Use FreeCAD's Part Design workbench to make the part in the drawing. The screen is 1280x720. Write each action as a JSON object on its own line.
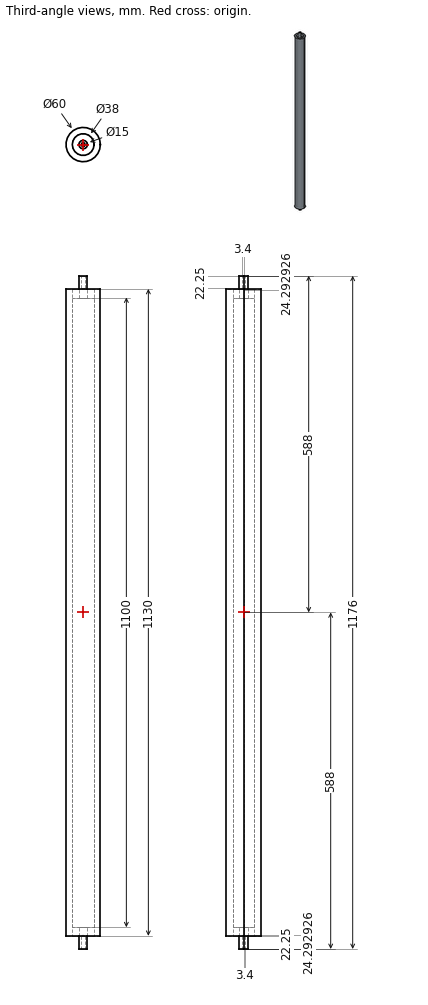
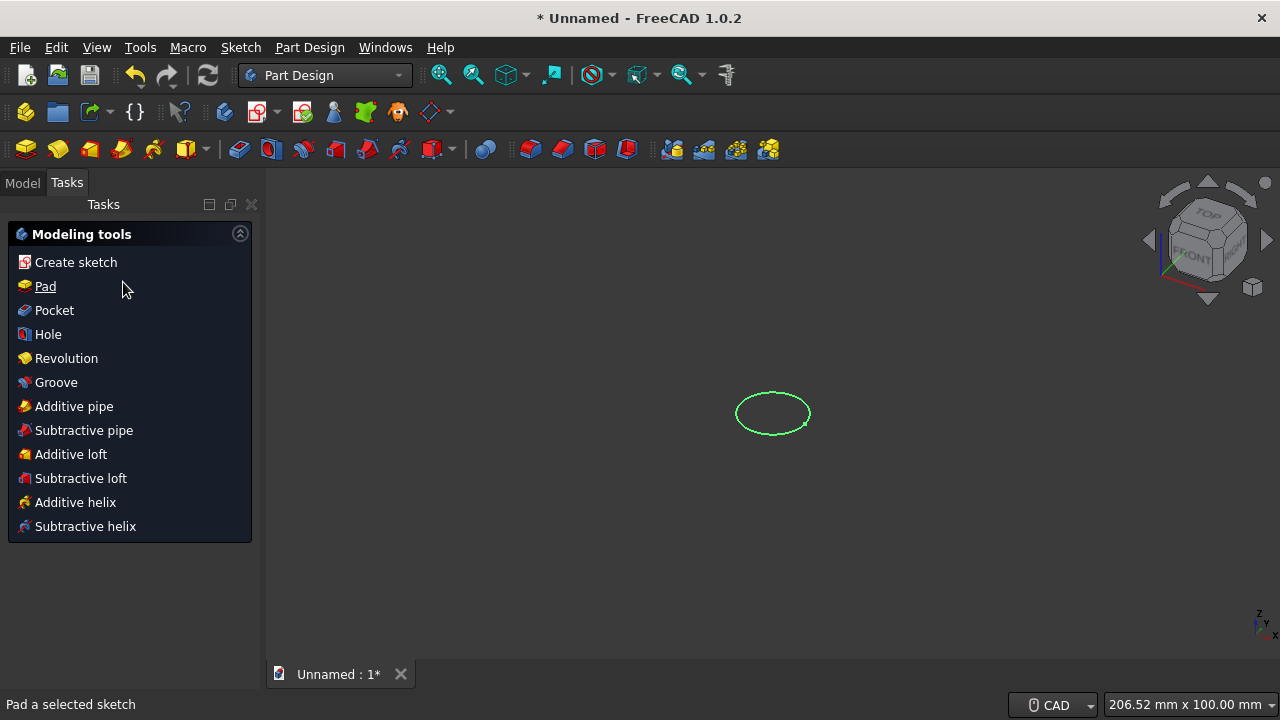
{"action": "left_click", "coordinate": [26, 150]}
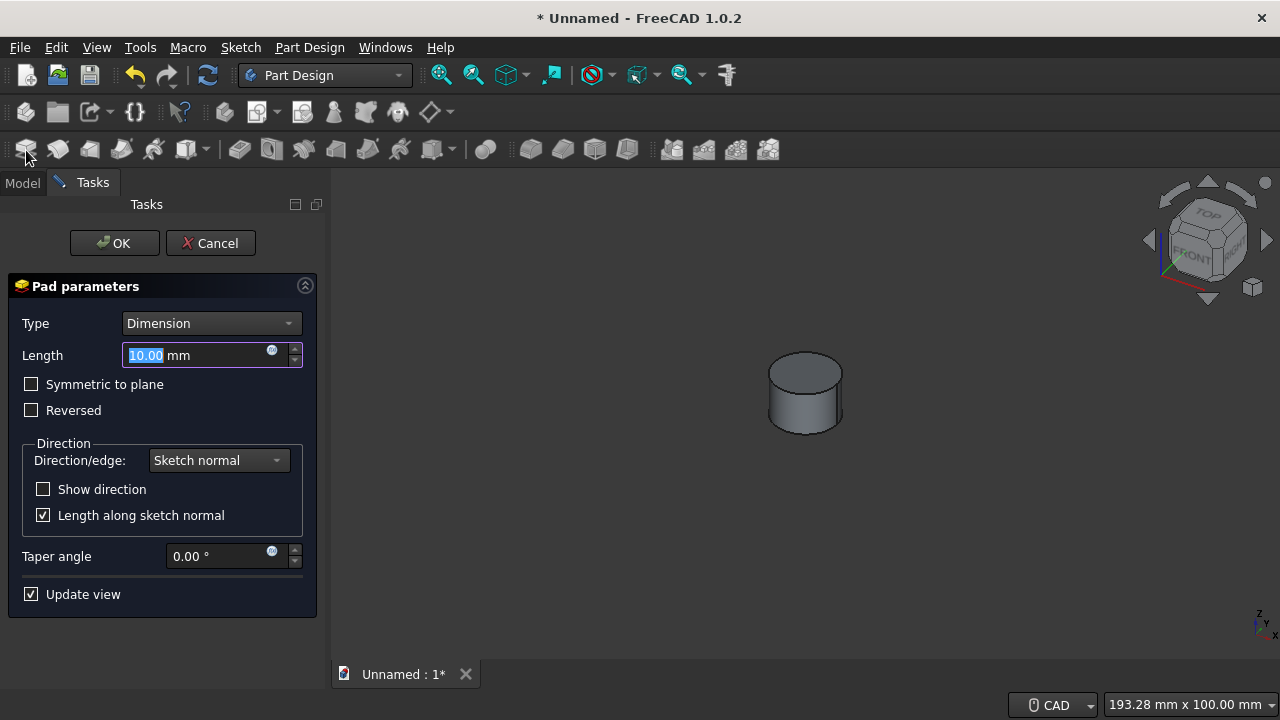
{"action": "type", "text": "1176"}
{"action": "key", "text": "Tab"}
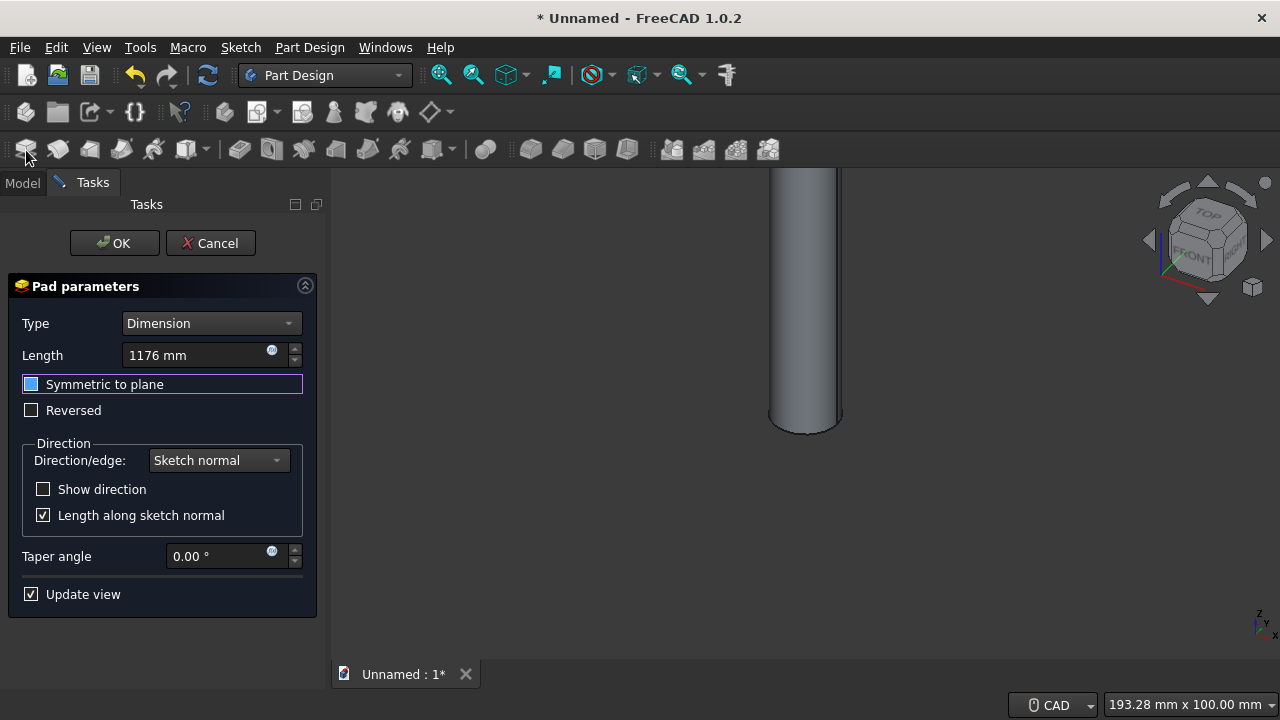
{"action": "left_click", "coordinate": [30, 384]}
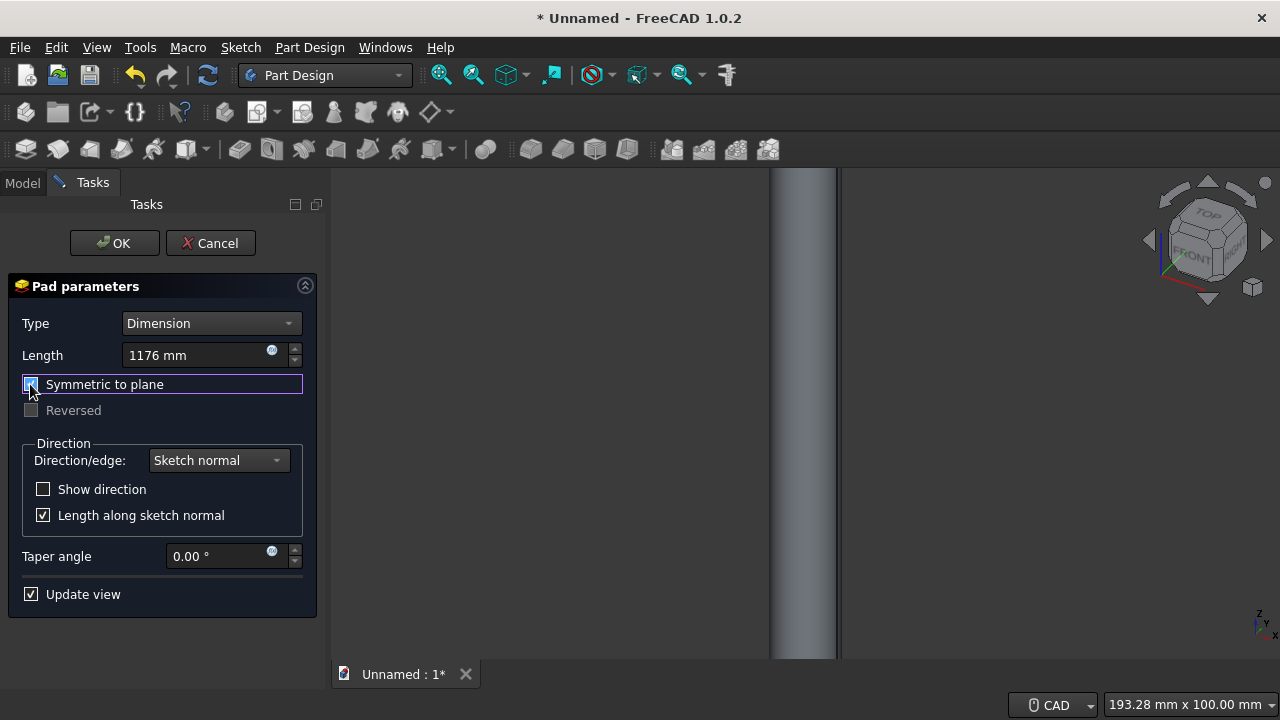
{"action": "left_click", "coordinate": [115, 243]}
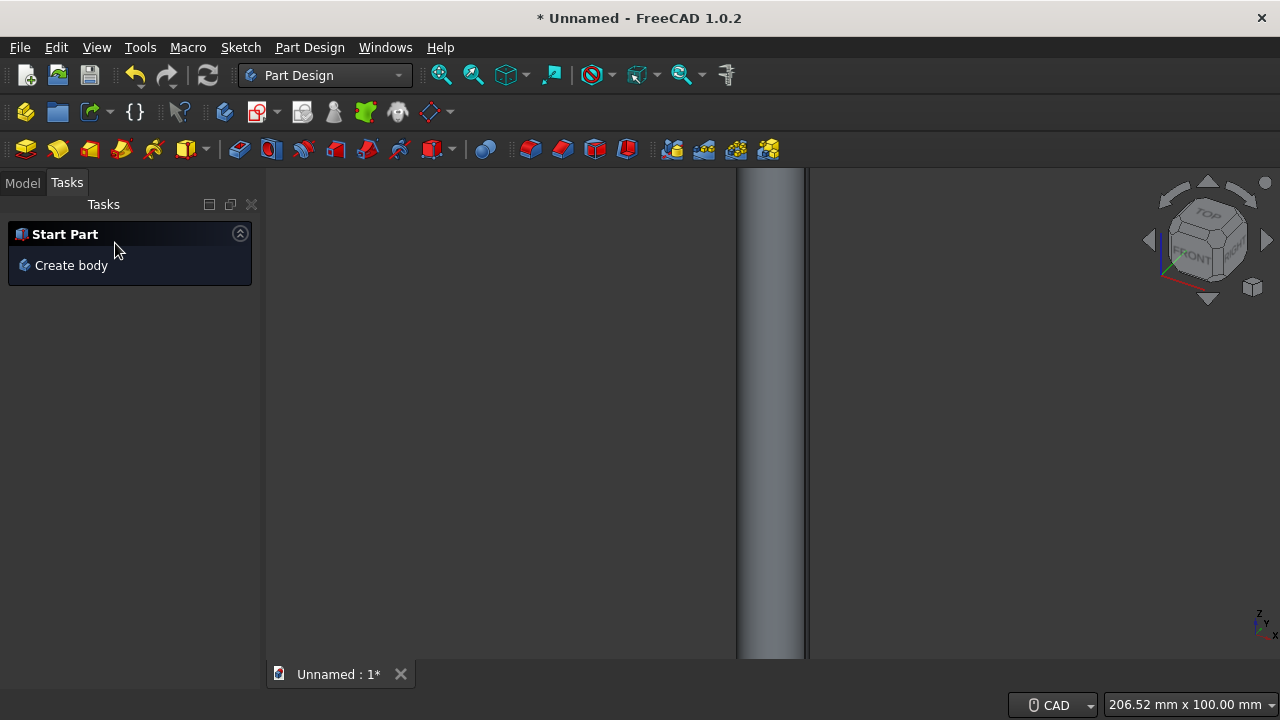
{"action": "left_click", "coordinate": [442, 76]}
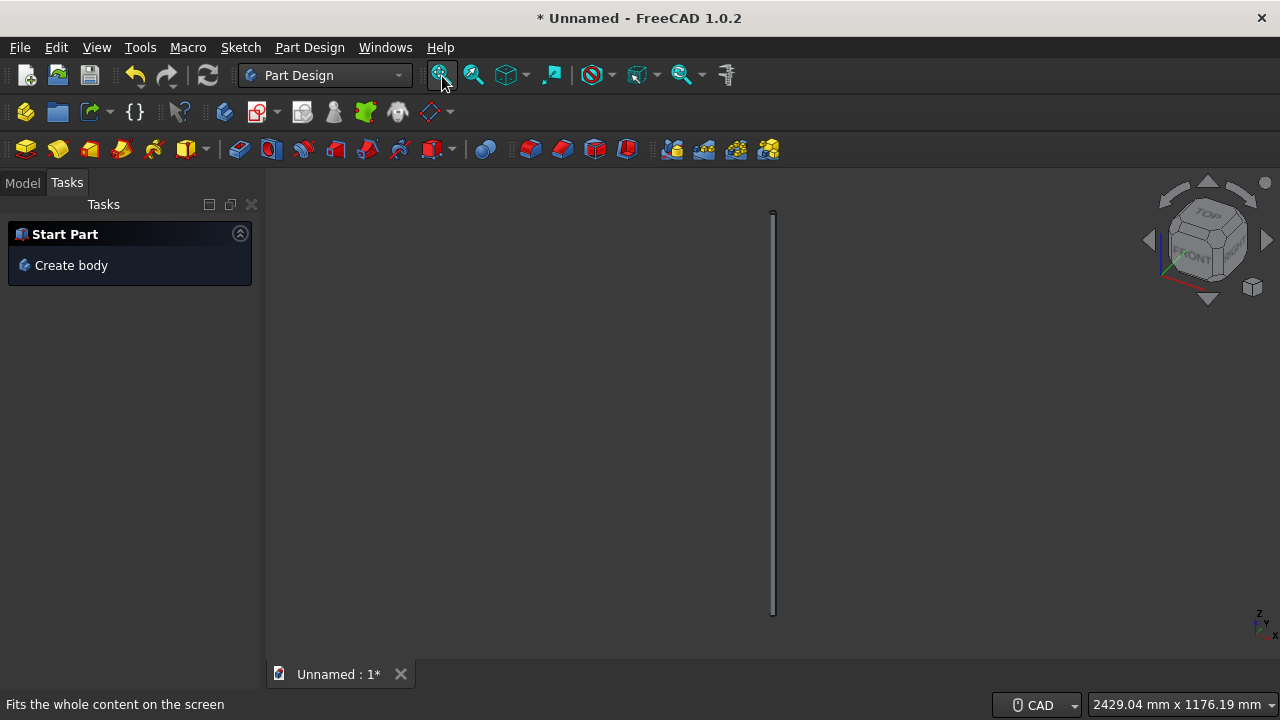
{"action": "left_click", "coordinate": [258, 112]}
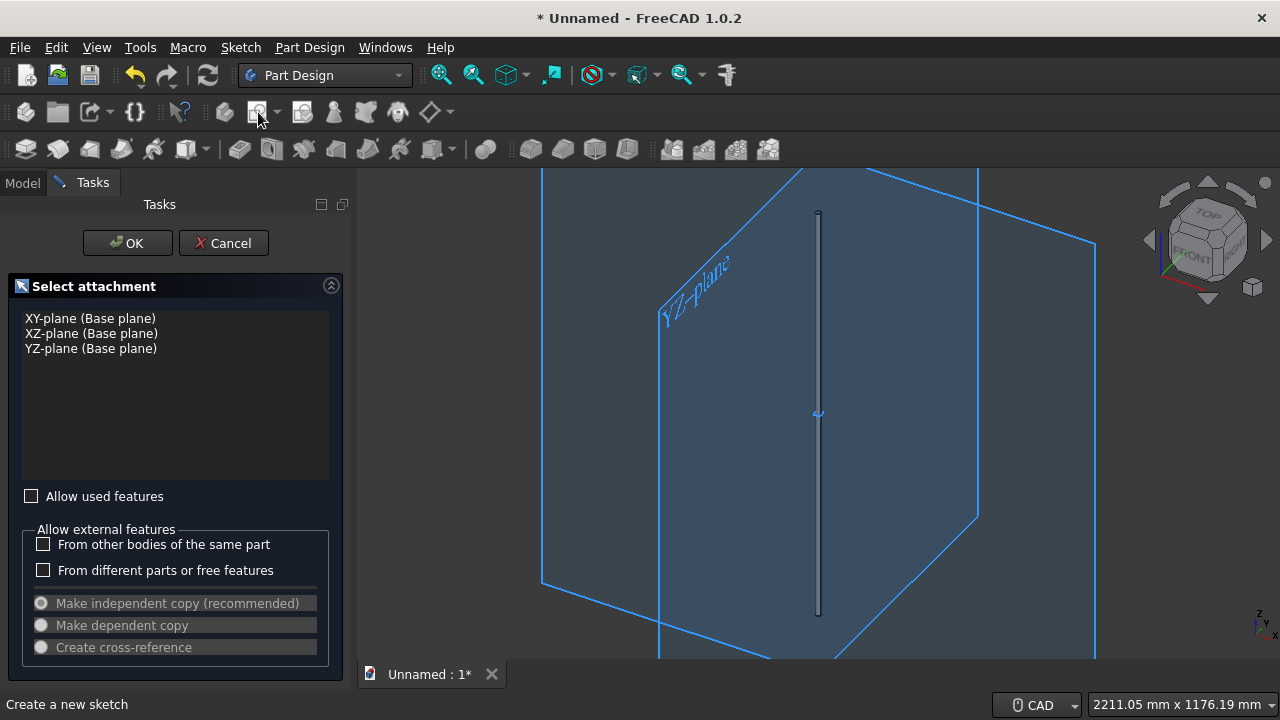
{"action": "left_click", "coordinate": [82, 318]}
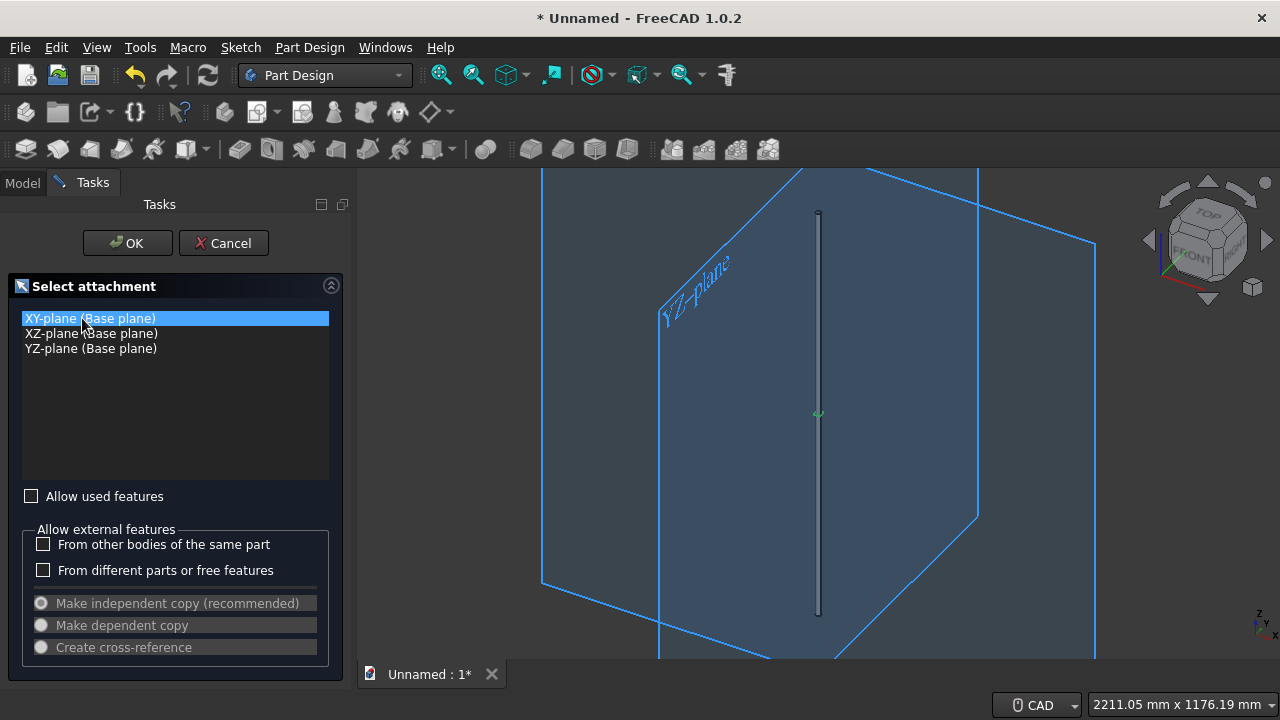
{"action": "left_click", "coordinate": [128, 243]}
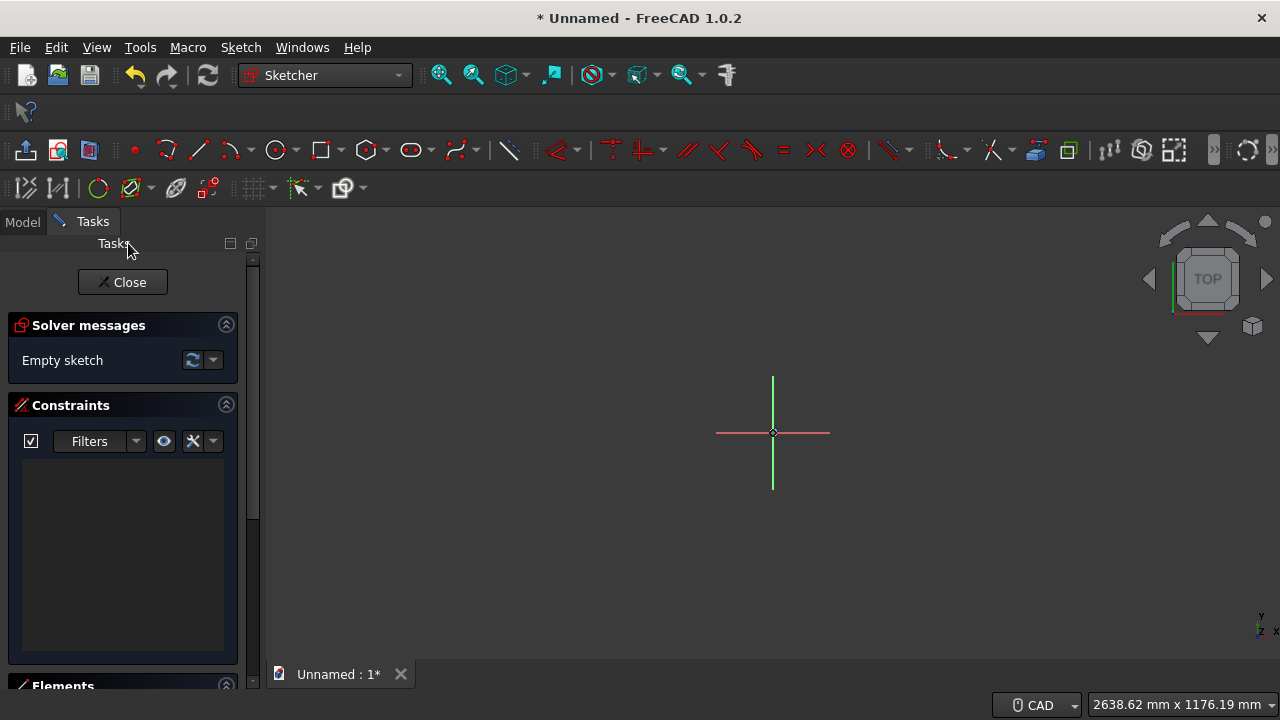
{"action": "left_click", "coordinate": [90, 150]}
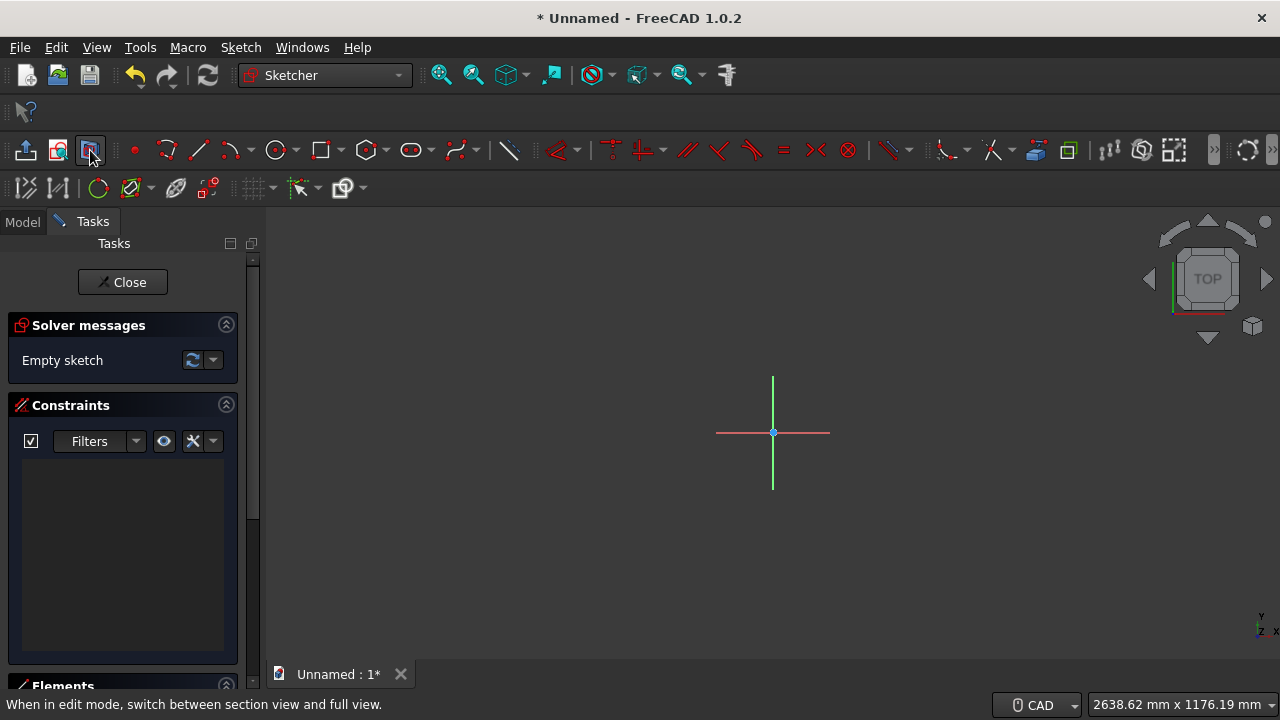
{"action": "scroll", "coordinate": [777, 433], "scroll_direction": "up", "scroll_amount": 15}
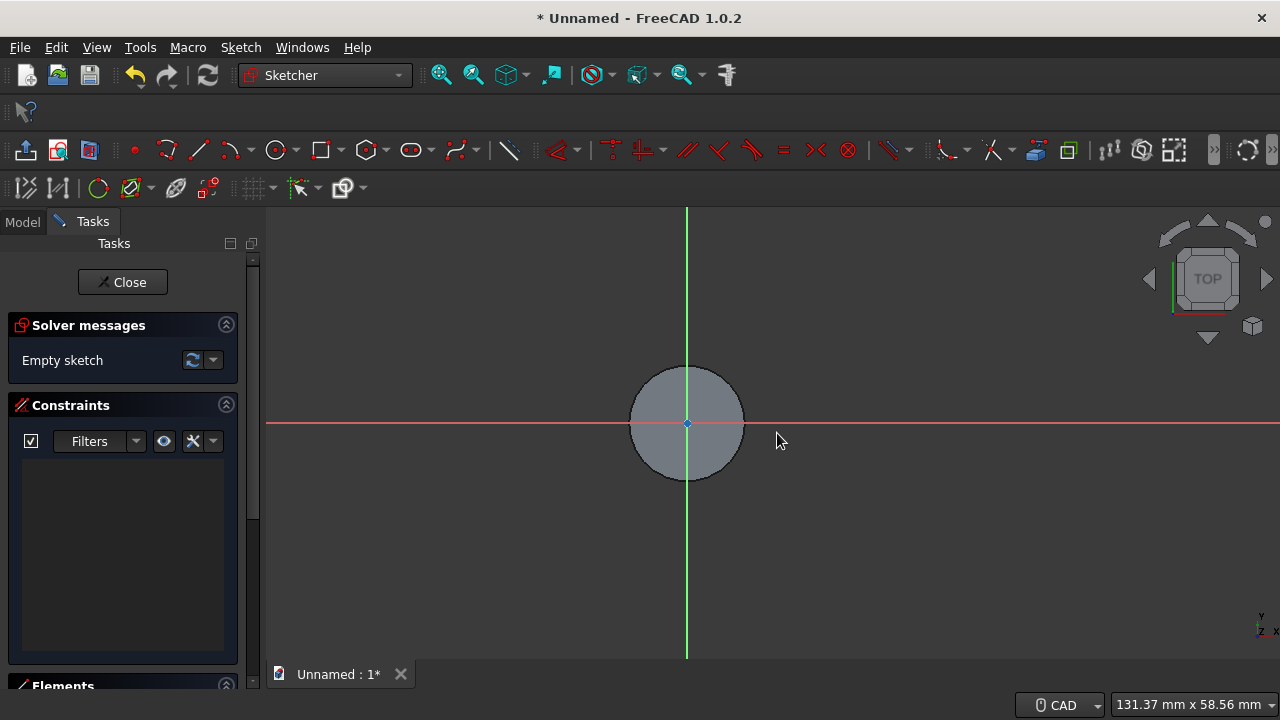
{"action": "key", "text": "g c"}